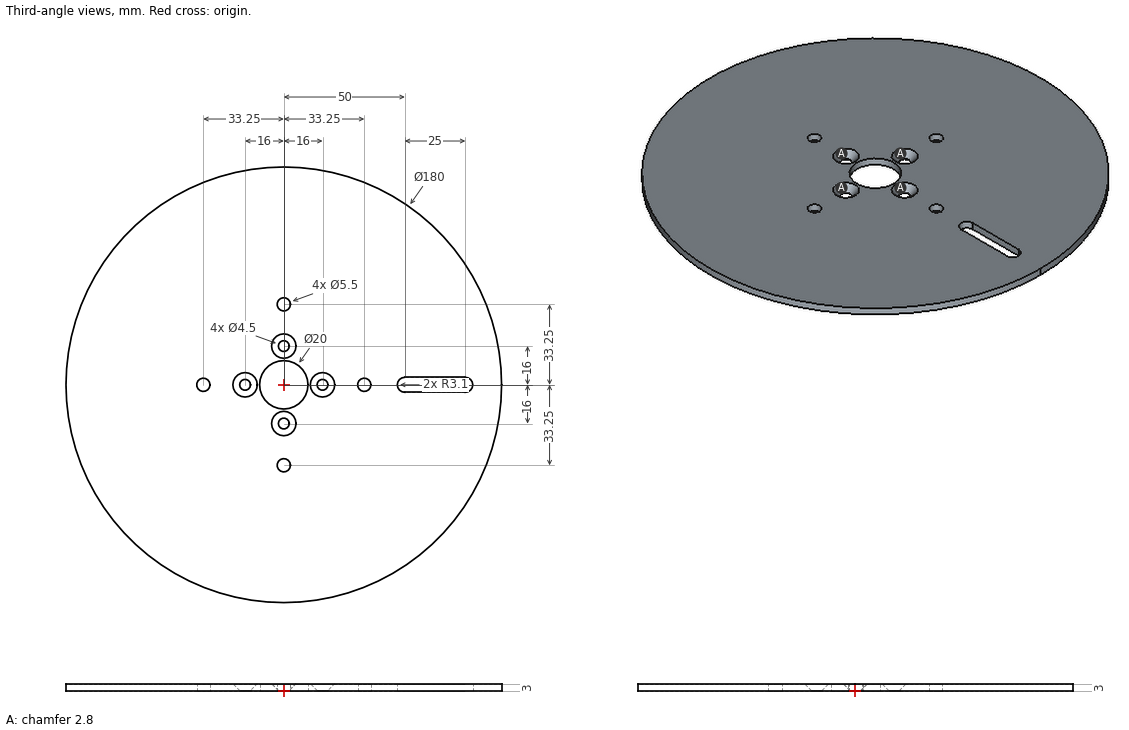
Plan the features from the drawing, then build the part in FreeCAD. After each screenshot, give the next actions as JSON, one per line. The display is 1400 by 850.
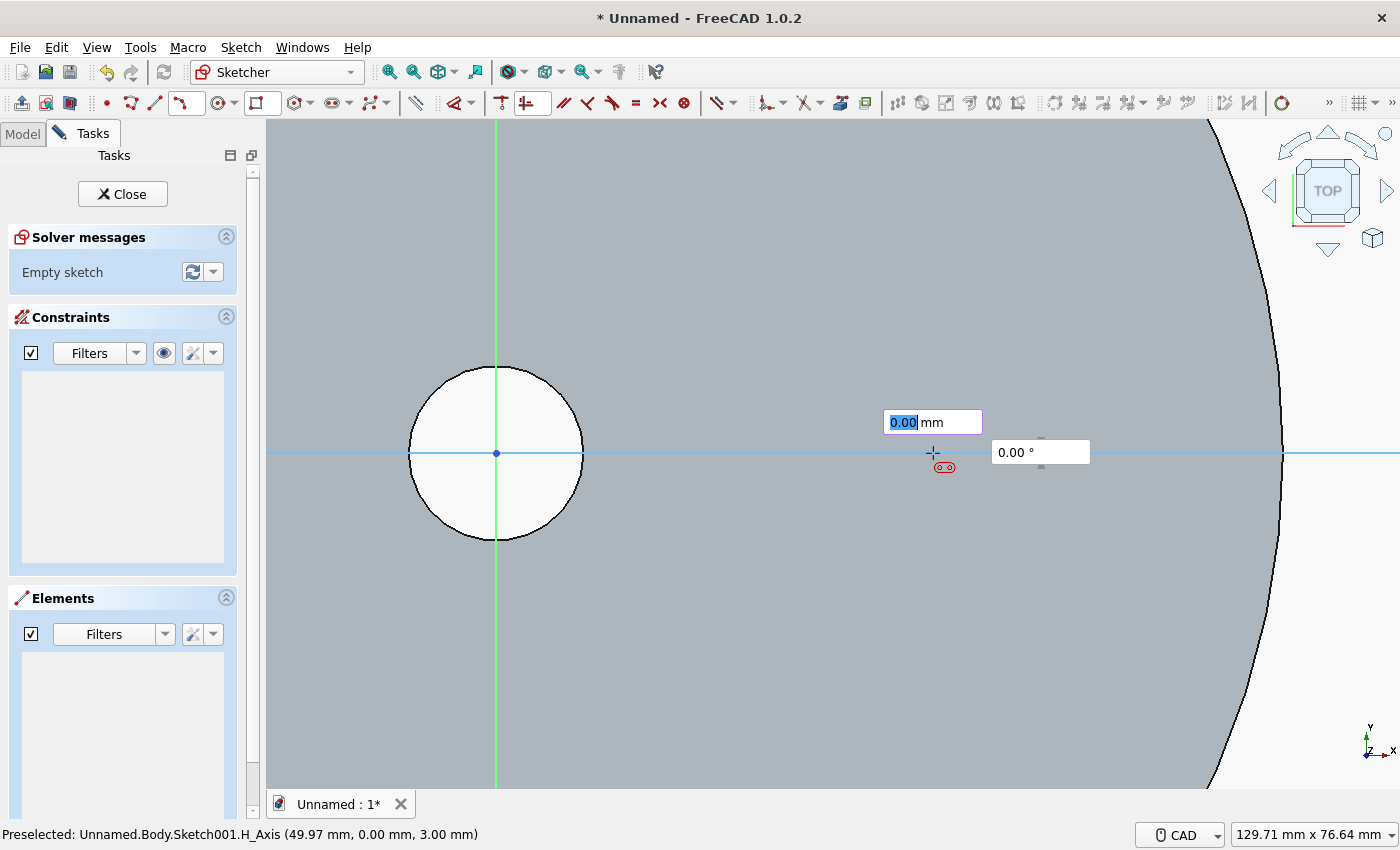
{"action": "left_click", "coordinate": [1152, 444]}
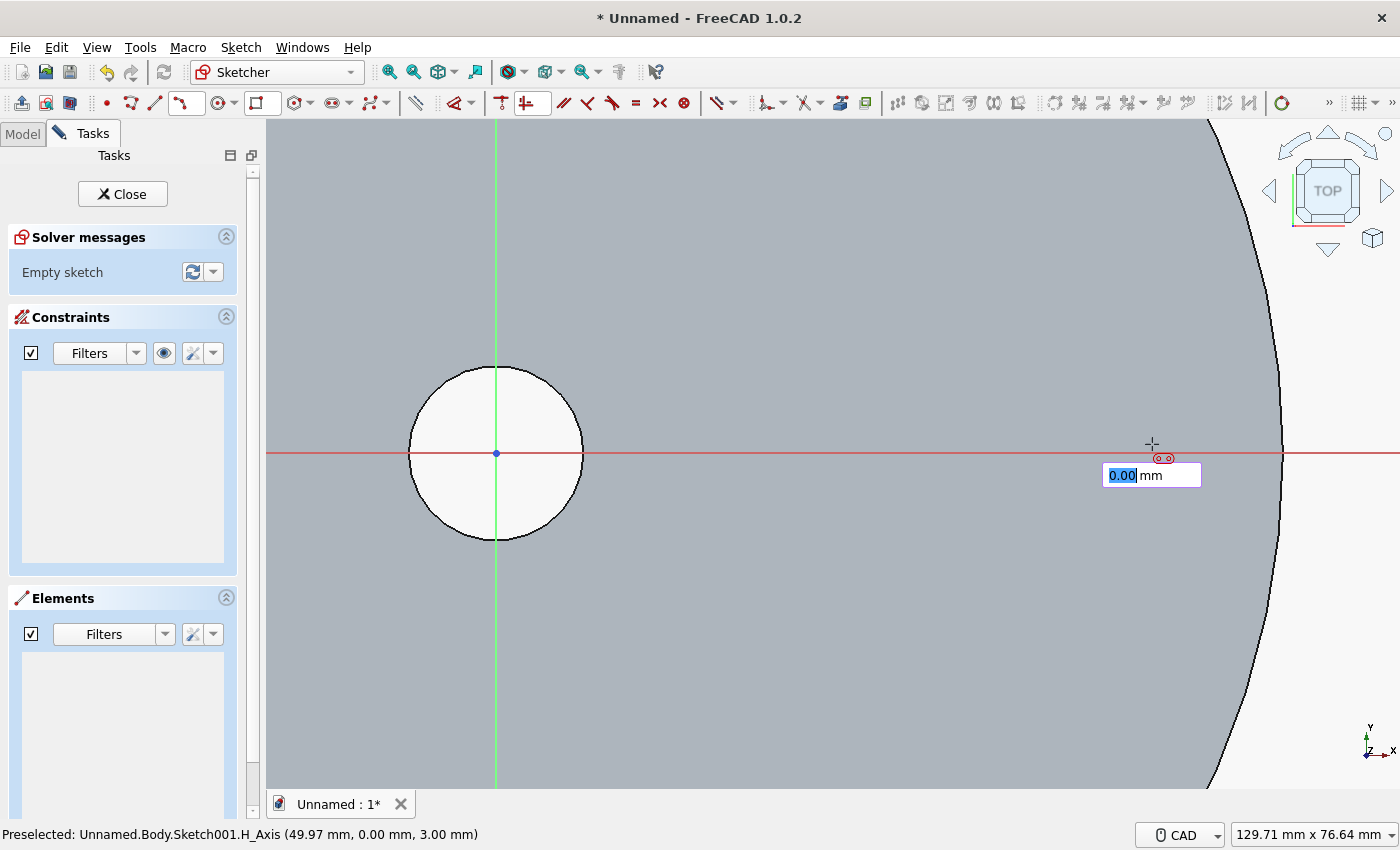
{"action": "left_click", "coordinate": [1043, 426]}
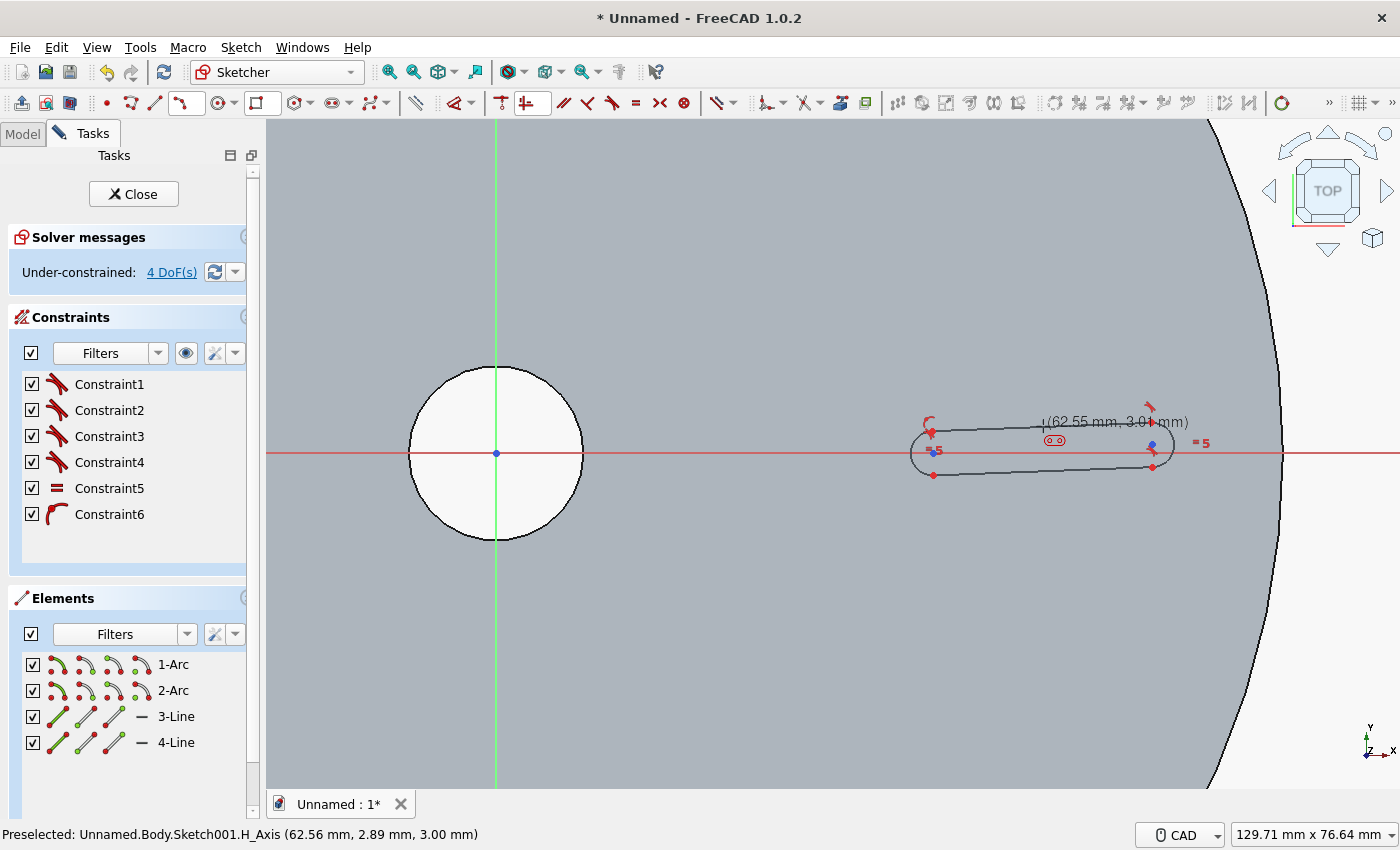
{"action": "left_click", "coordinate": [218, 104]}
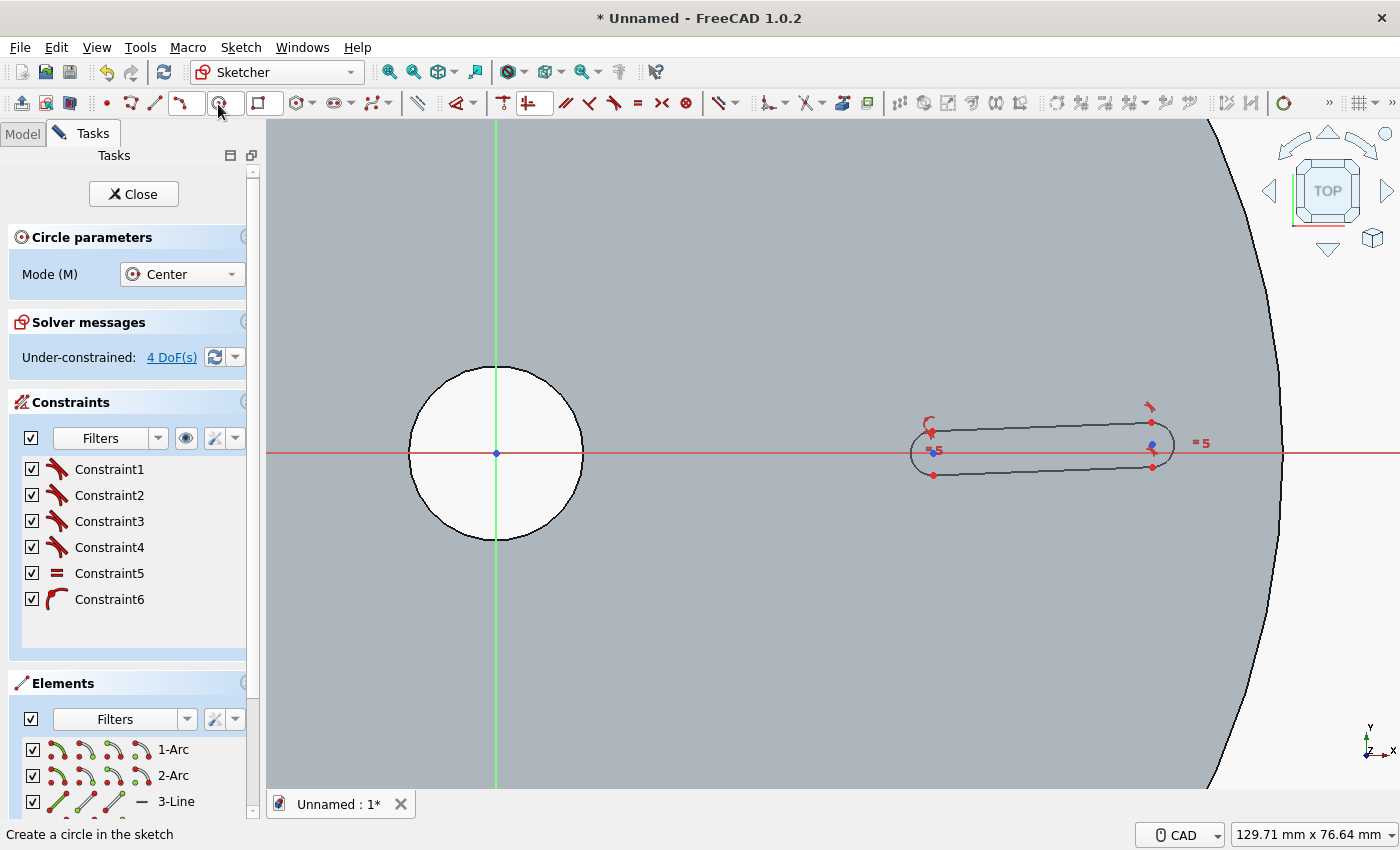
{"action": "left_click", "coordinate": [496, 313]}
{"action": "left_click", "coordinate": [515, 307]}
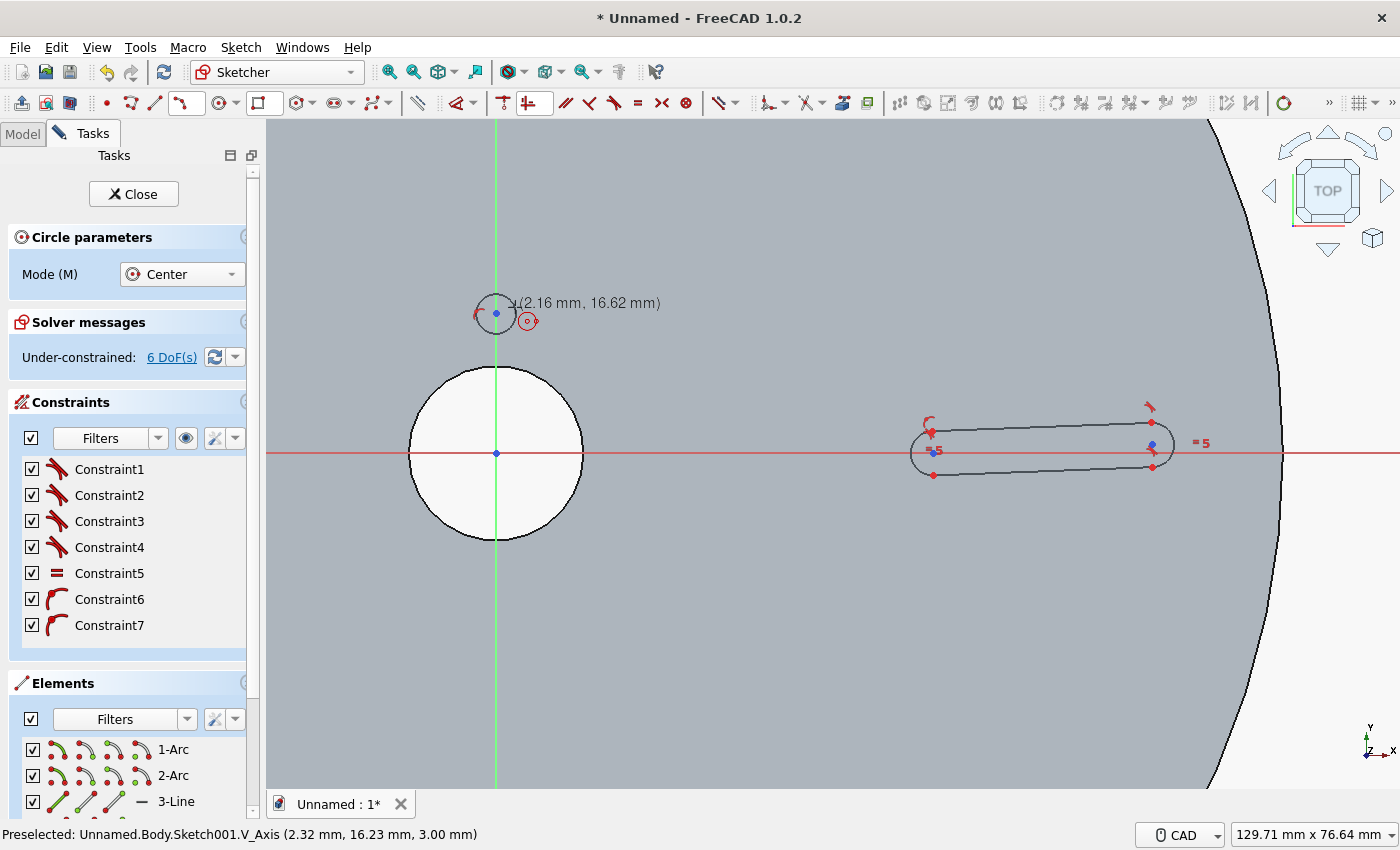
{"action": "left_click", "coordinate": [356, 453]}
{"action": "left_click", "coordinate": [363, 435]}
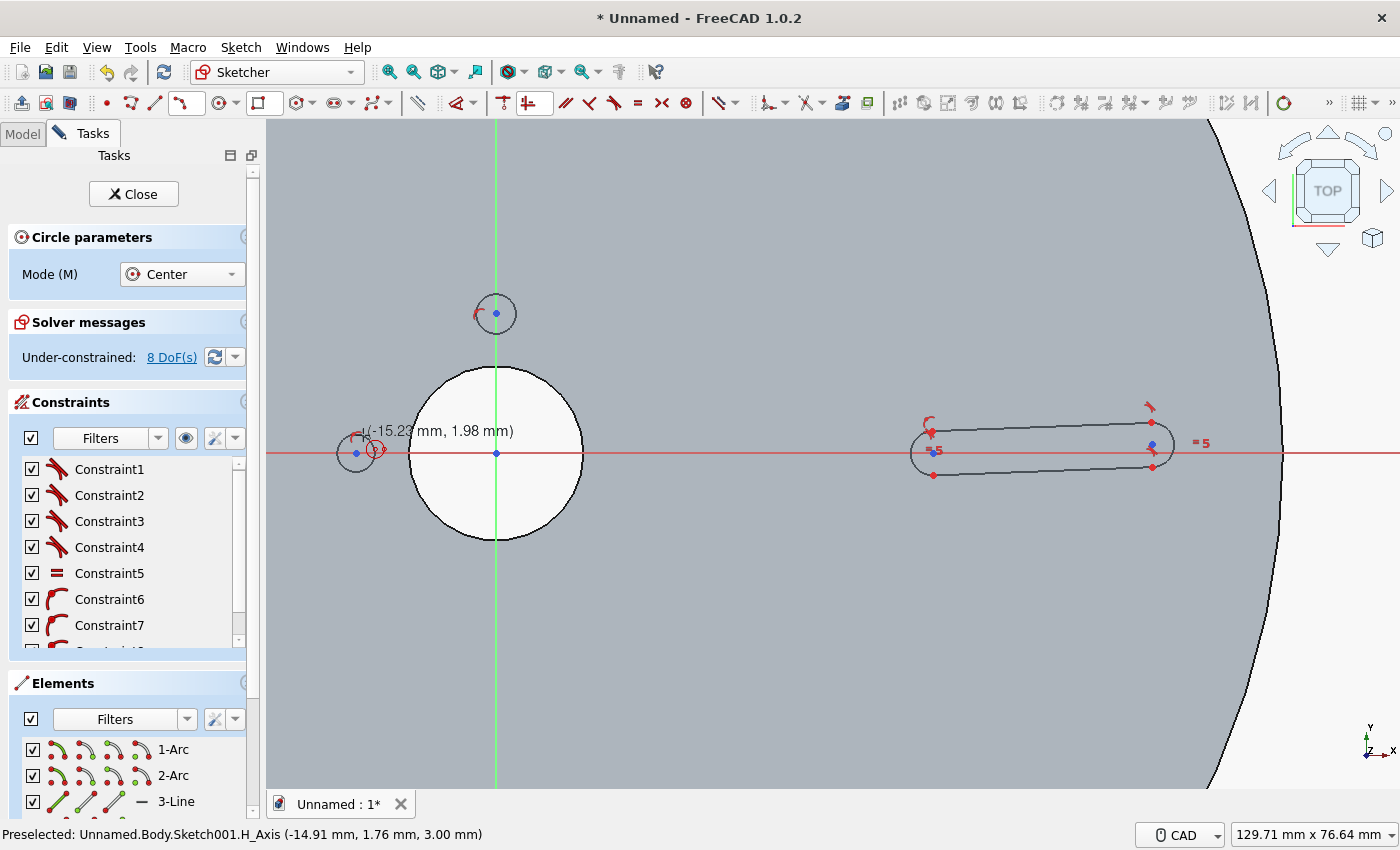
{"action": "left_click", "coordinate": [496, 593]}
{"action": "left_click", "coordinate": [515, 586]}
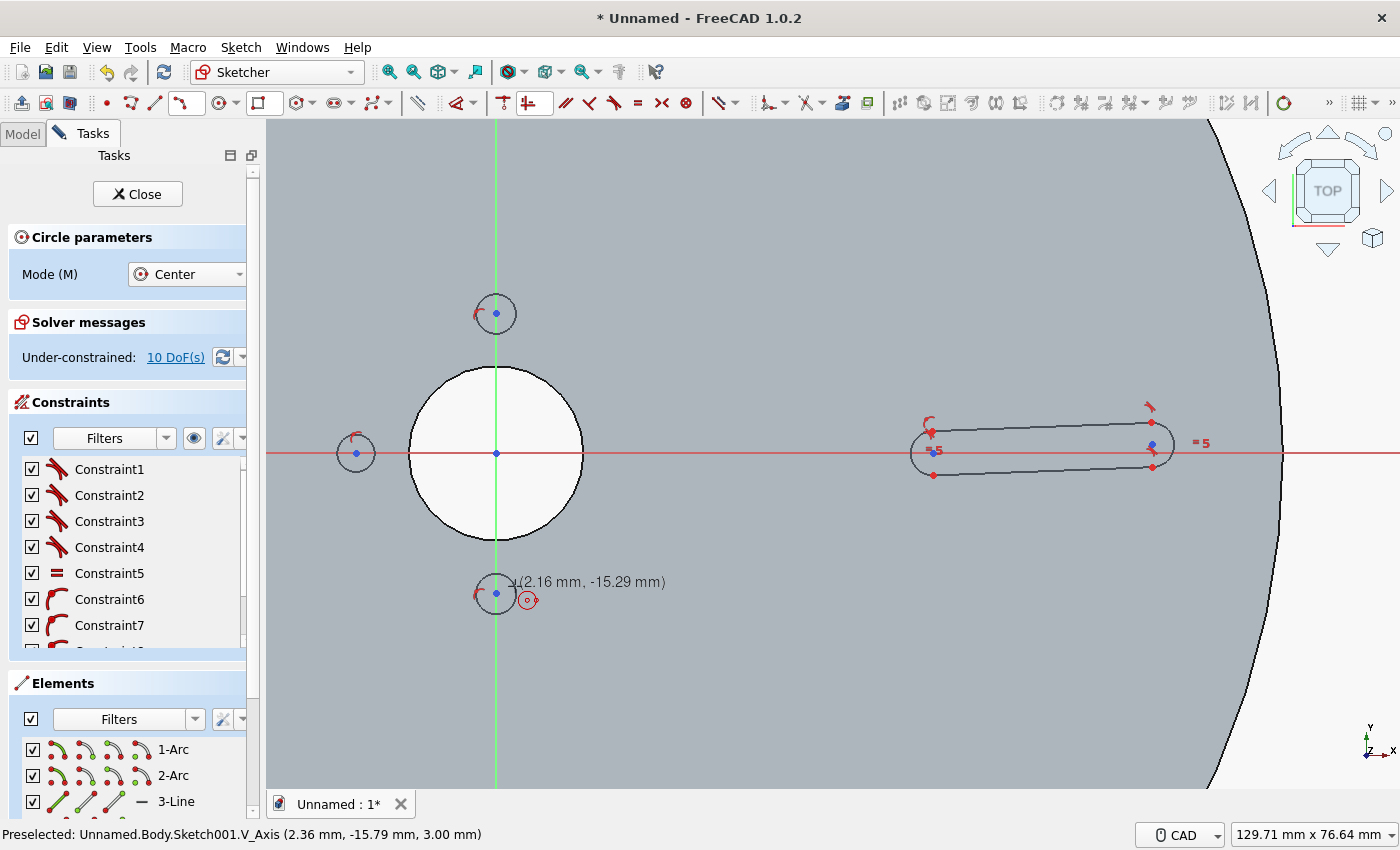
{"action": "left_click", "coordinate": [636, 453]}
{"action": "left_click", "coordinate": [643, 435]}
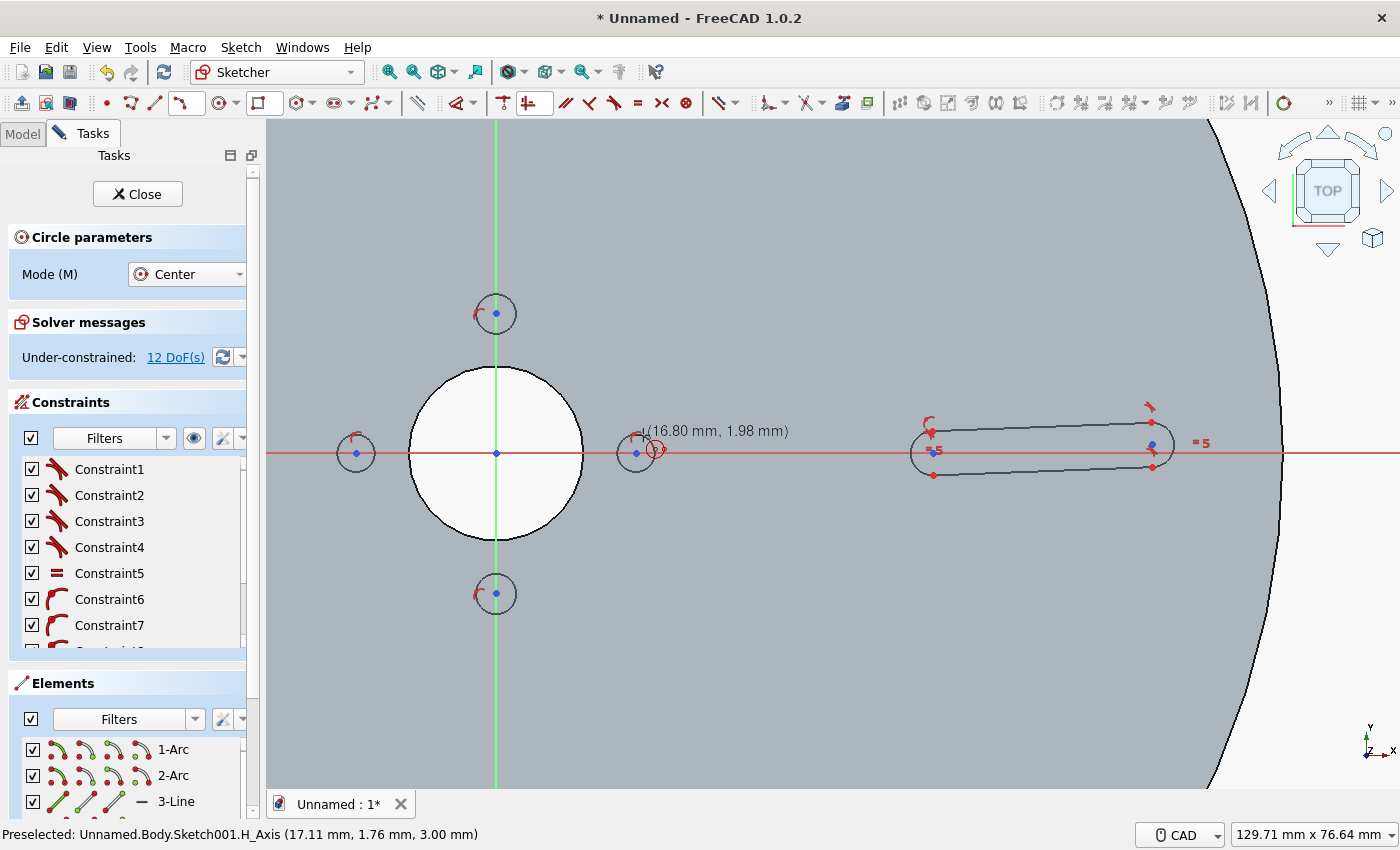
{"action": "left_click", "coordinate": [496, 163]}